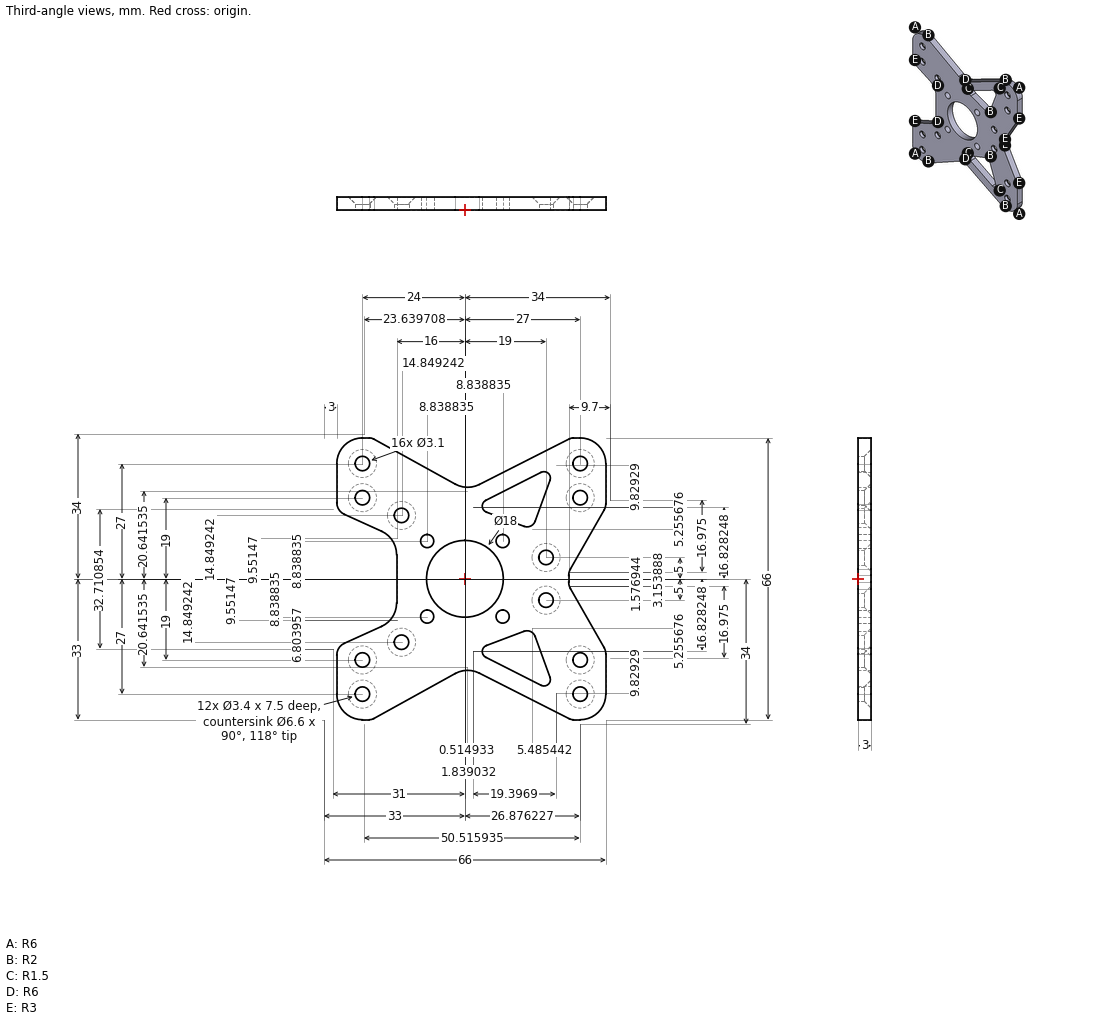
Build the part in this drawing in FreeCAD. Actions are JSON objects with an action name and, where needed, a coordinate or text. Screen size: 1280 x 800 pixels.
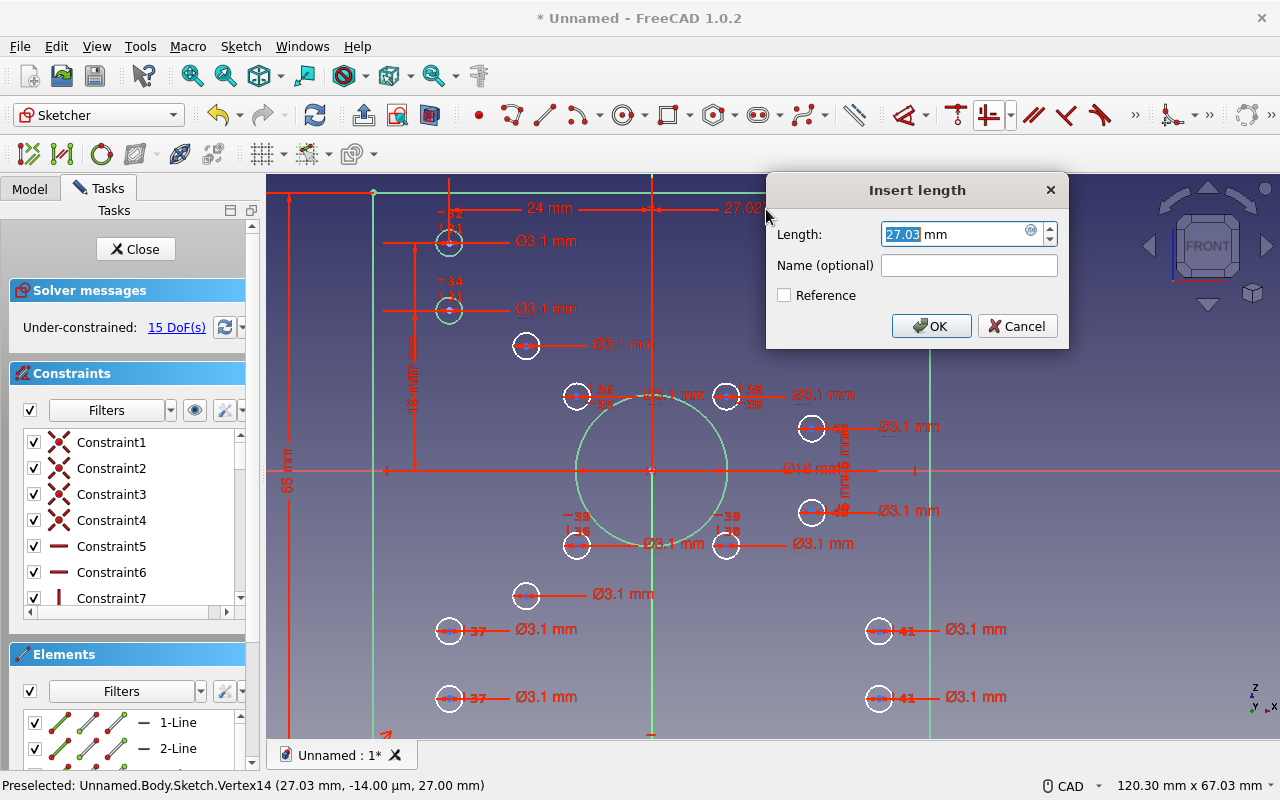
{"action": "type", "text": "27"}
{"action": "key", "text": "Return"}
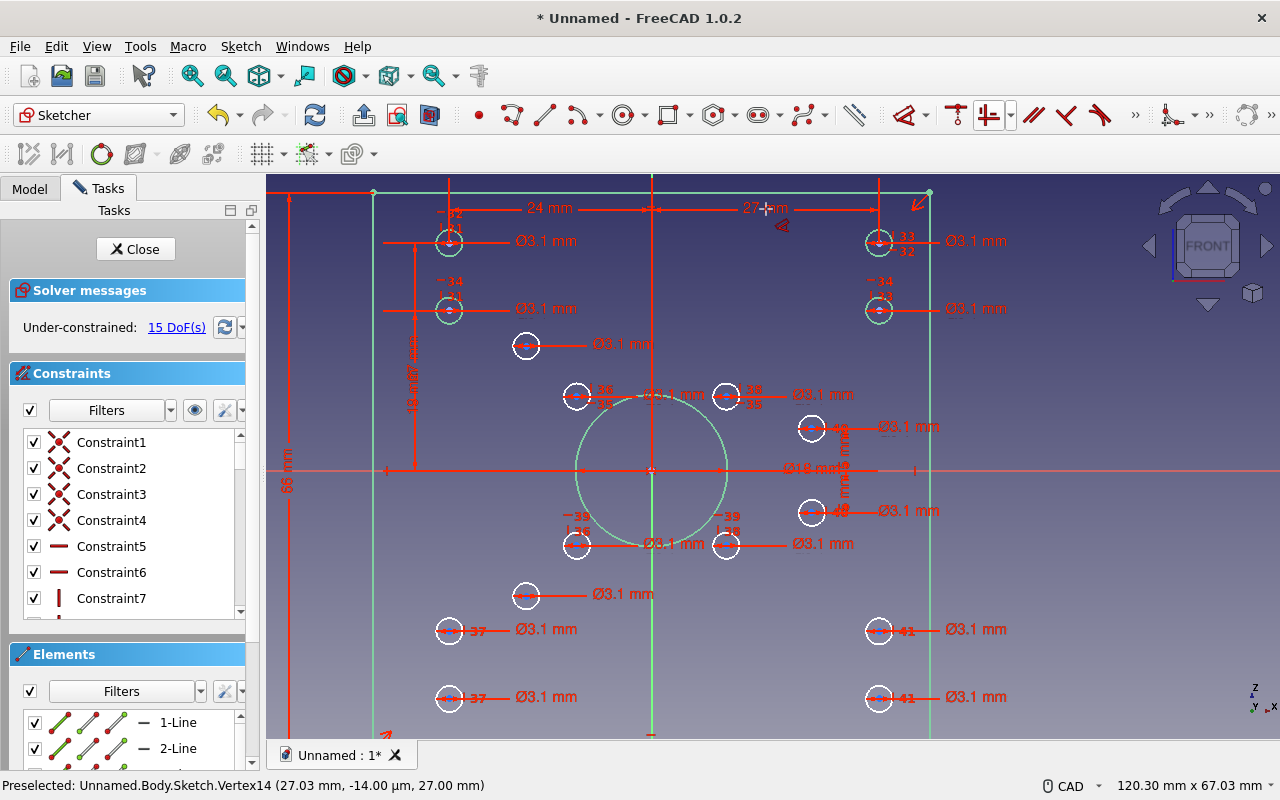
{"action": "left_click", "coordinate": [812, 429]}
{"action": "left_click", "coordinate": [769, 395]}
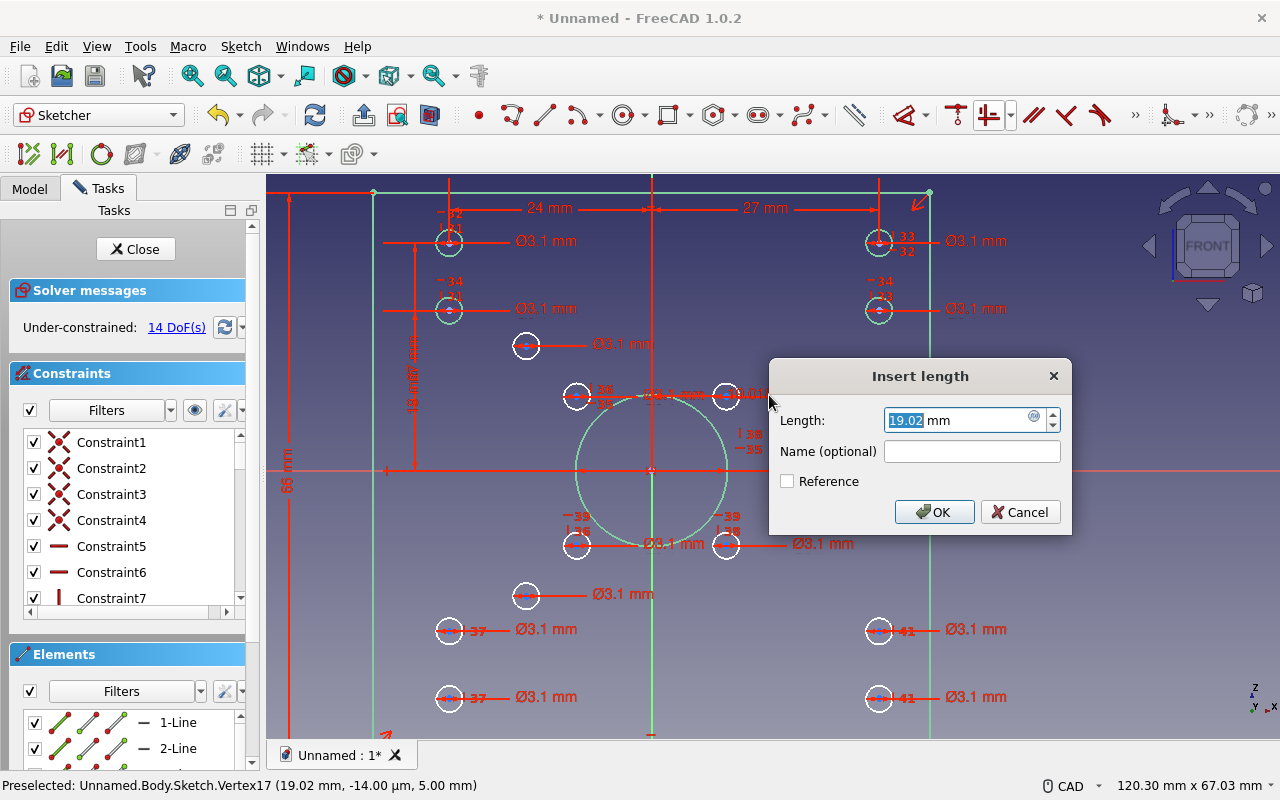
{"action": "type", "text": "19"}
{"action": "key", "text": "Return"}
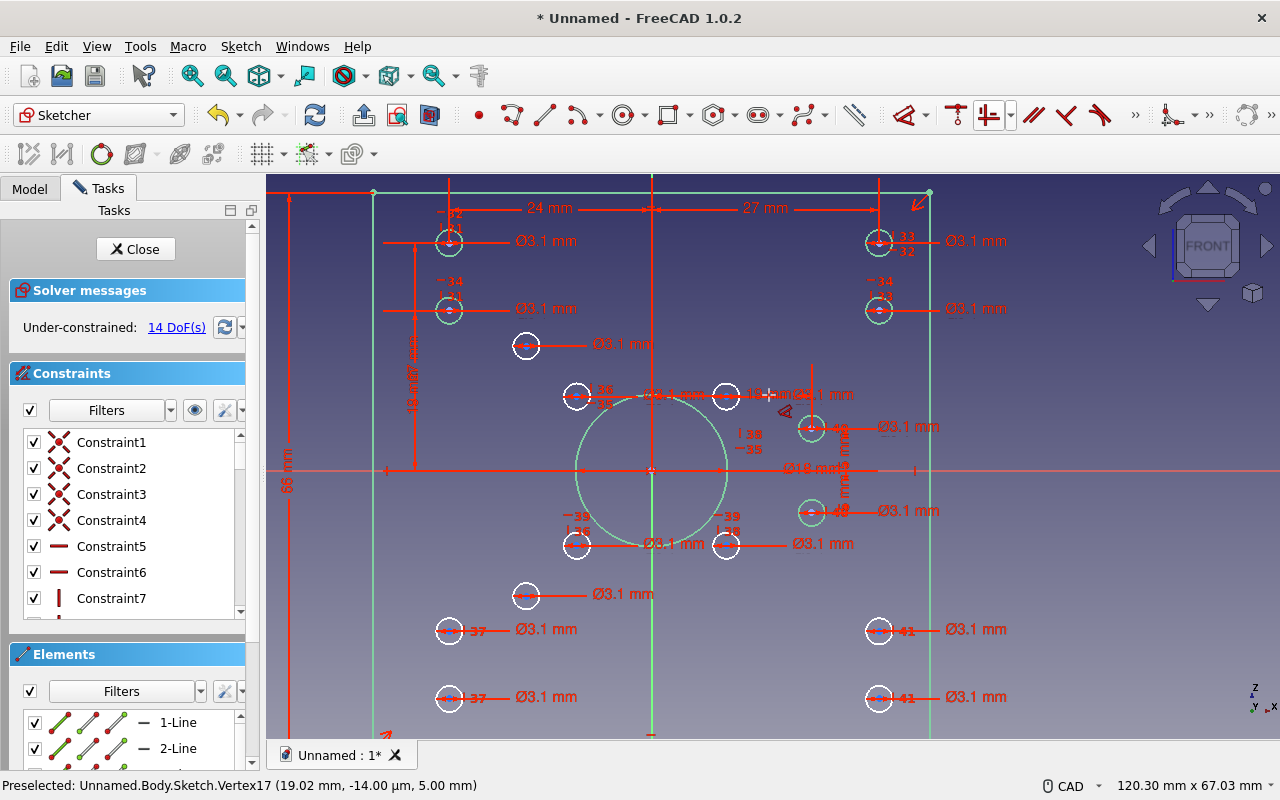
{"action": "left_click", "coordinate": [449, 631]}
{"action": "left_click", "coordinate": [551, 665]}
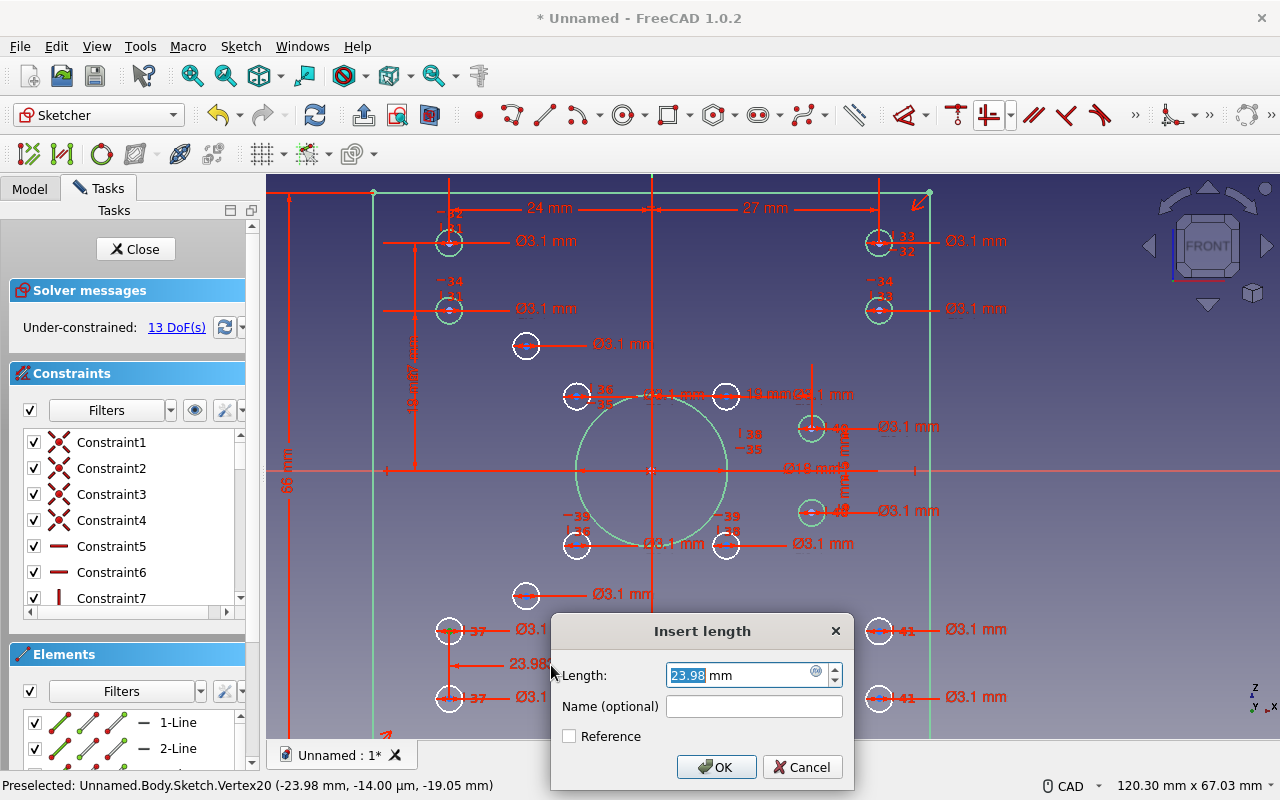
{"action": "type", "text": "24"}
{"action": "key", "text": "Return"}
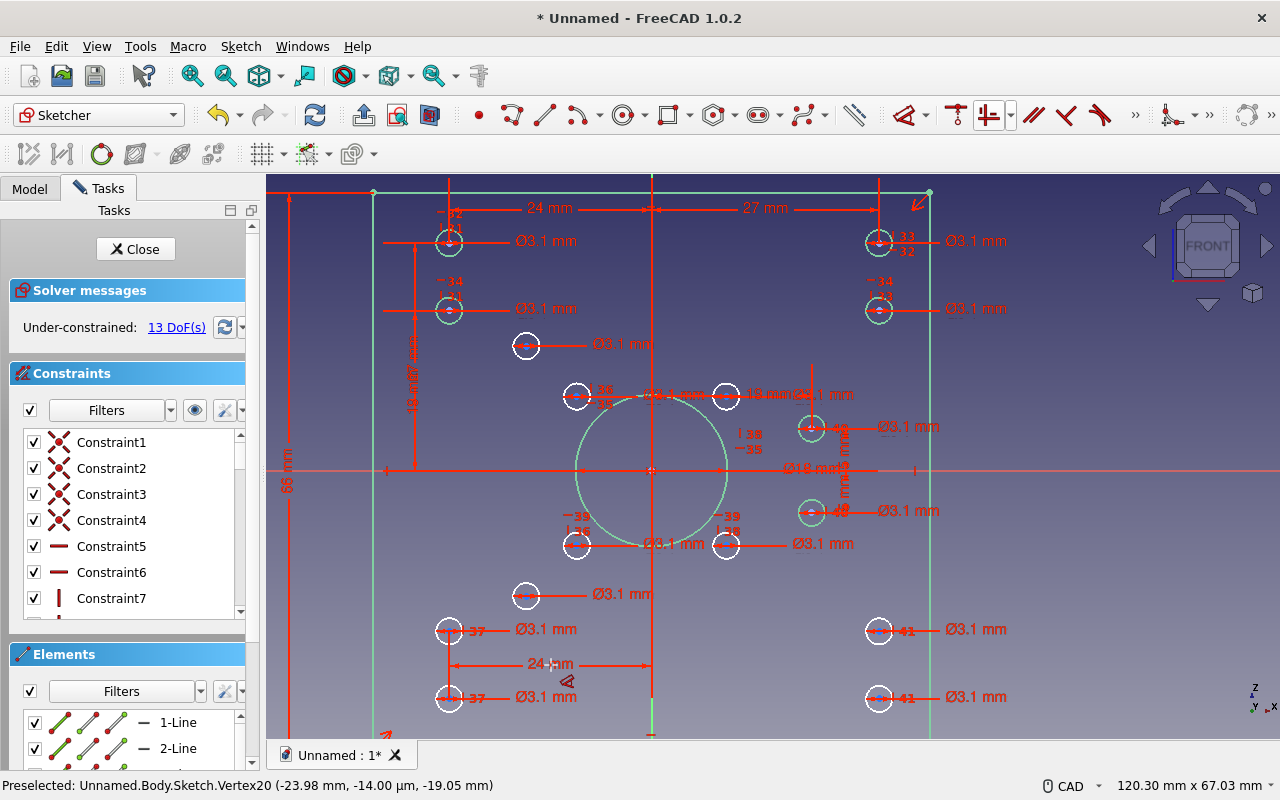
{"action": "left_click", "coordinate": [449, 631]}
{"action": "left_click", "coordinate": [415, 551]}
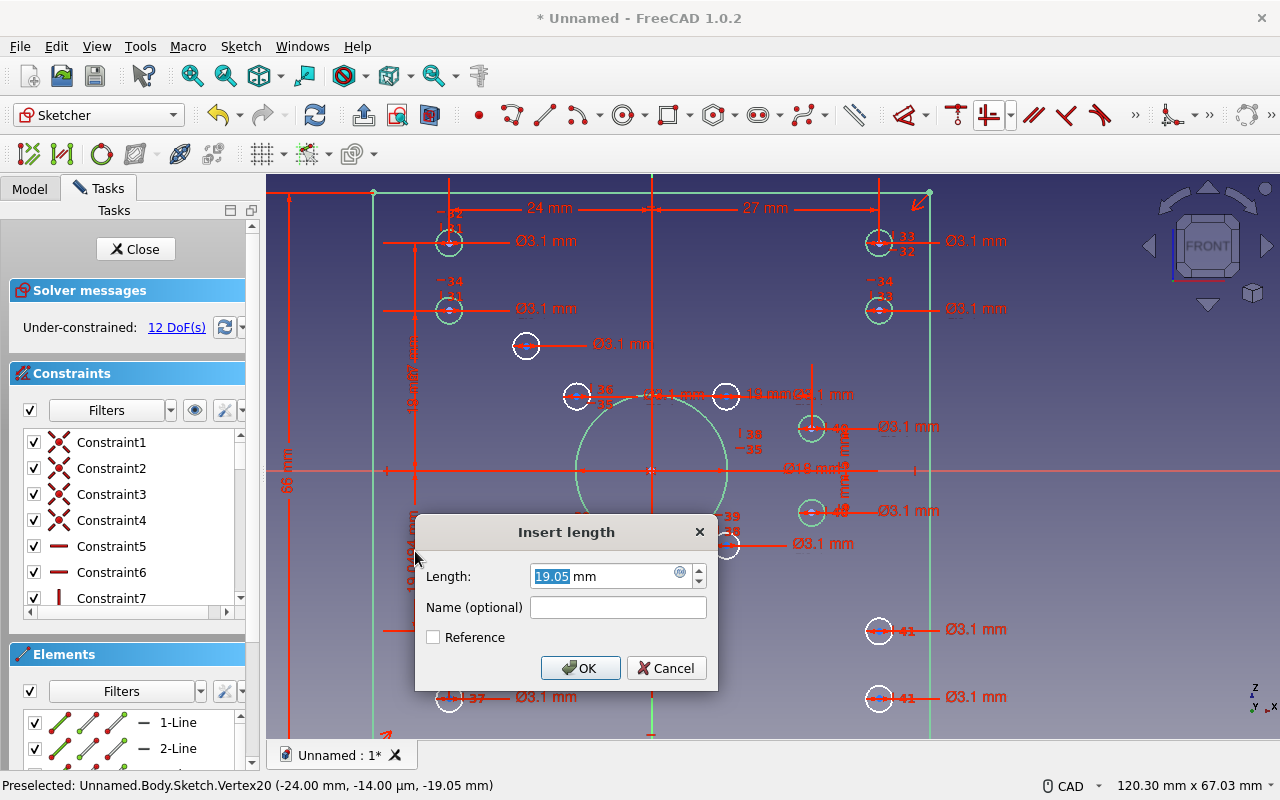
{"action": "type", "text": "19"}
{"action": "key", "text": "Return"}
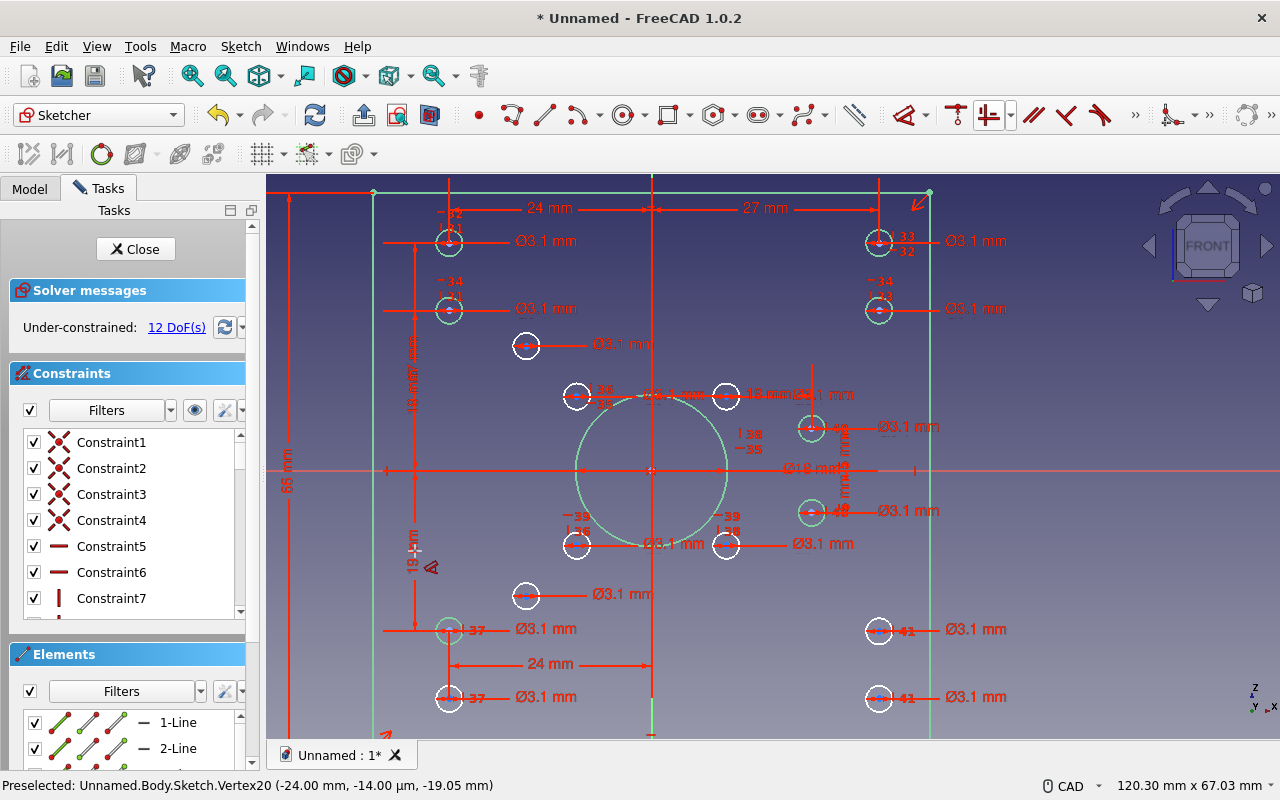
{"action": "left_click", "coordinate": [449, 699]}
{"action": "left_click", "coordinate": [415, 585]}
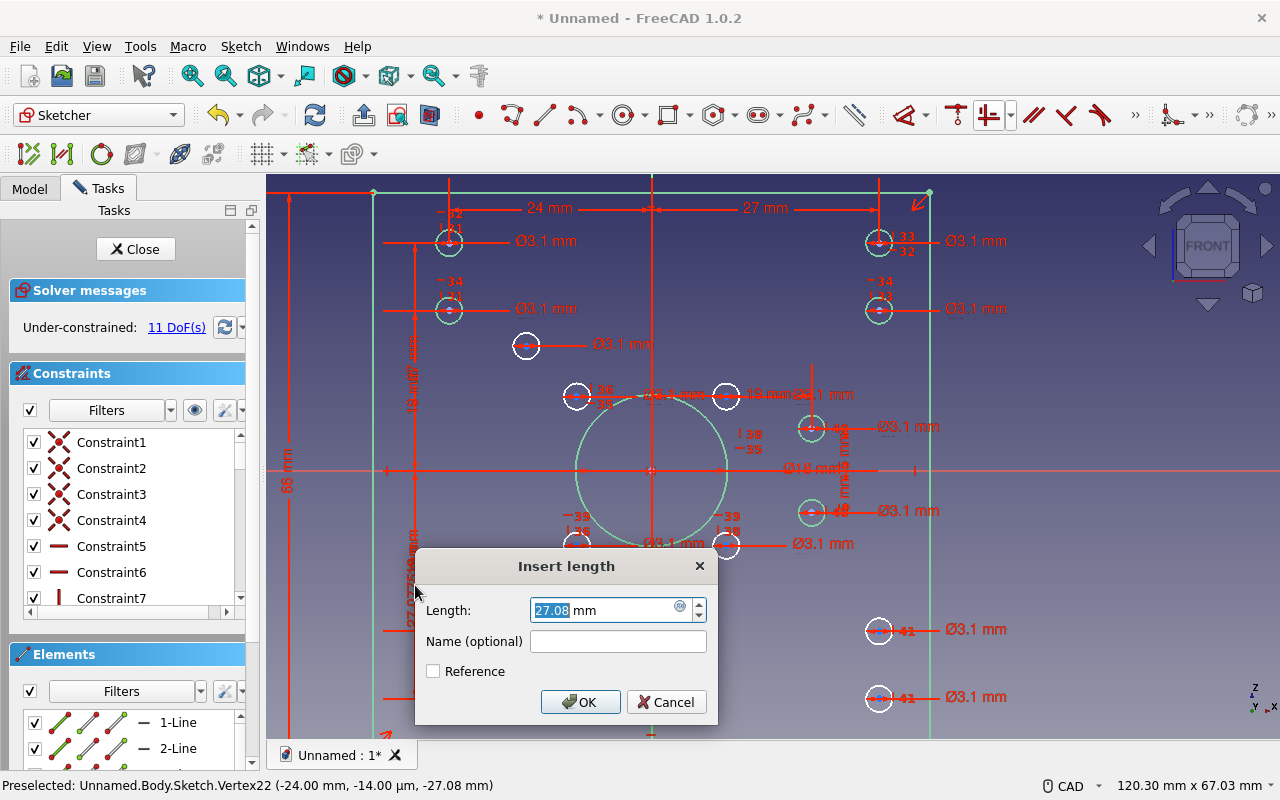
{"action": "type", "text": "27"}
{"action": "key", "text": "Return"}